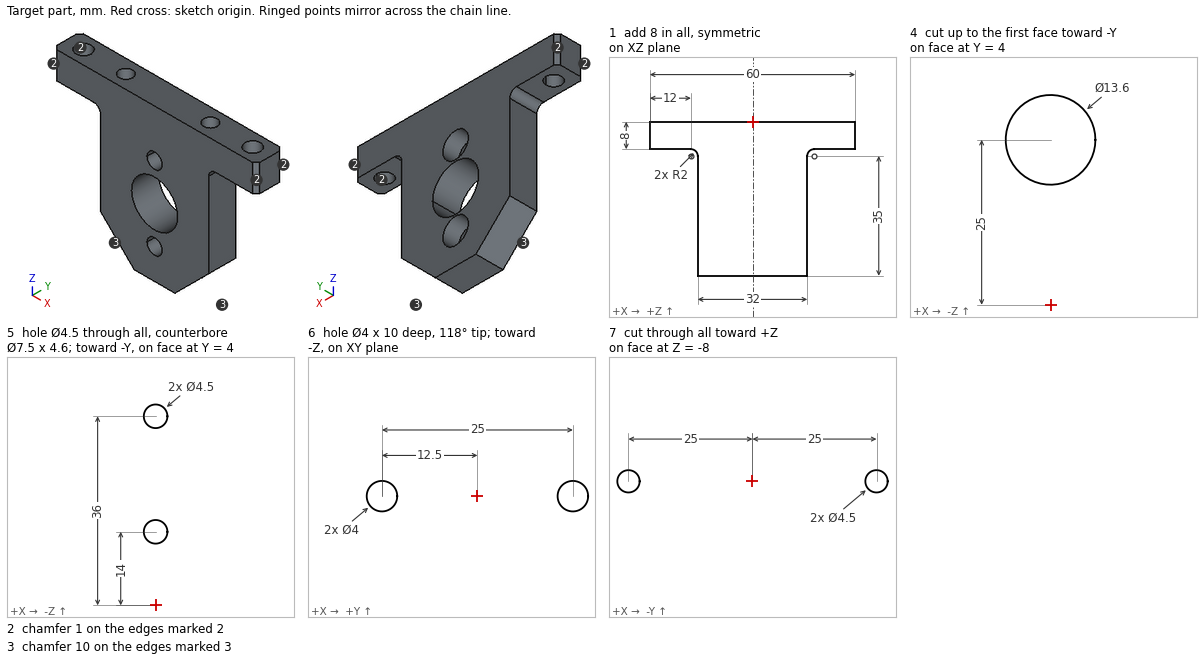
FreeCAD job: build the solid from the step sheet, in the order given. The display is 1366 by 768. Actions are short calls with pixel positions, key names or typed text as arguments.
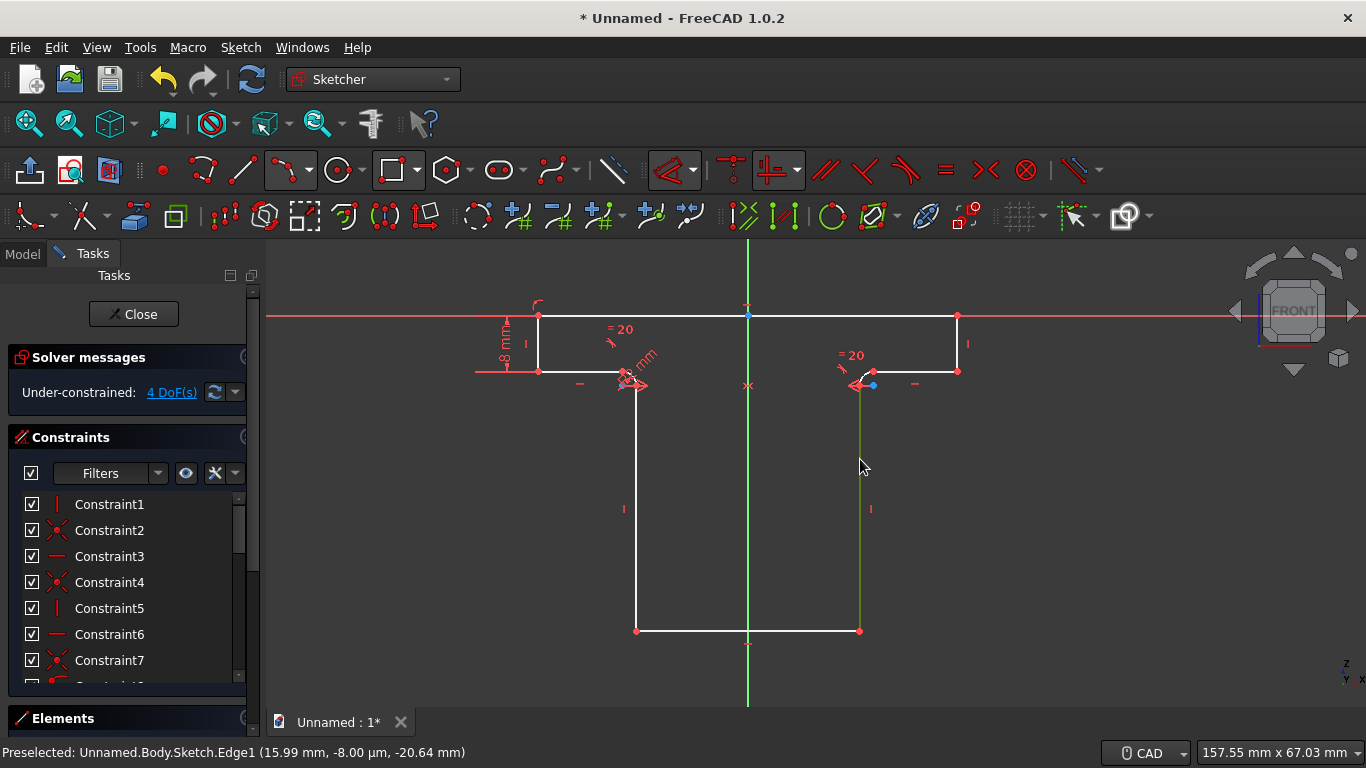
click(696, 170)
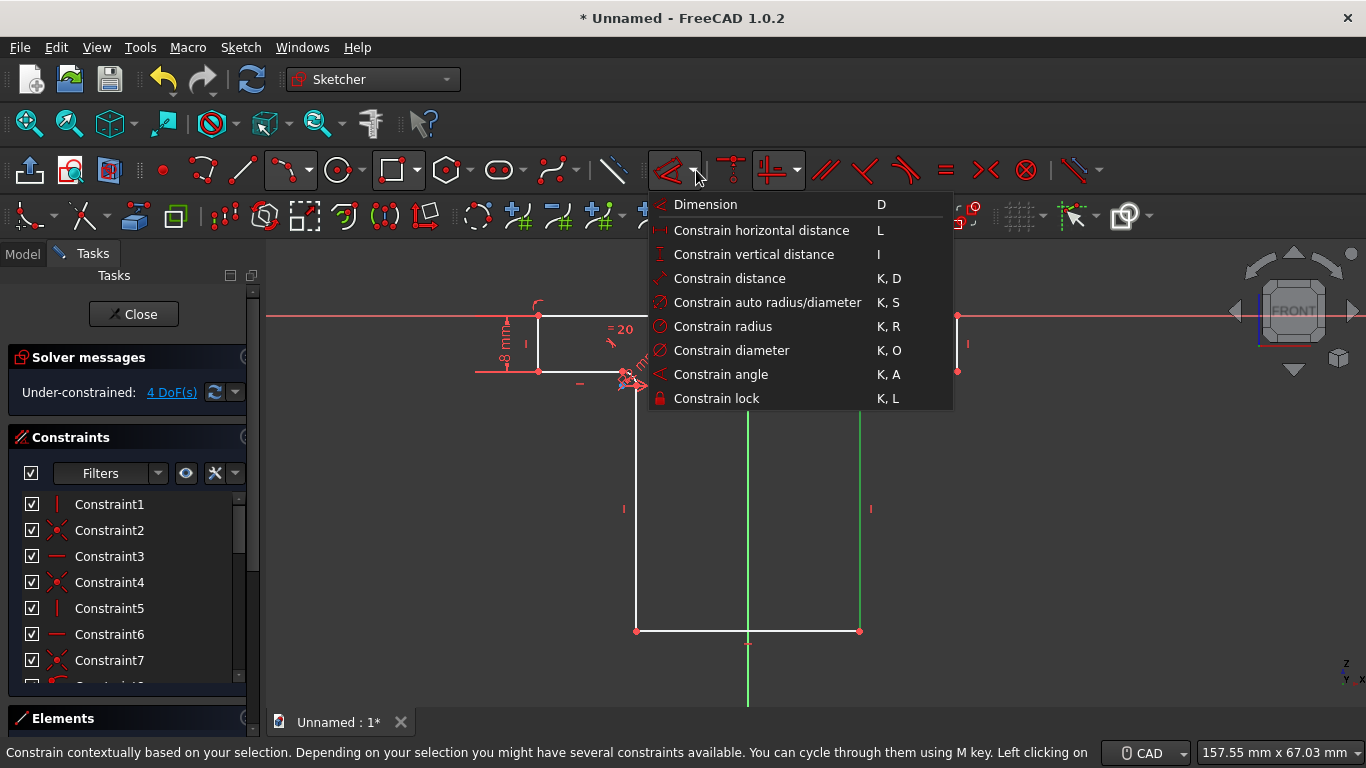
click(801, 254)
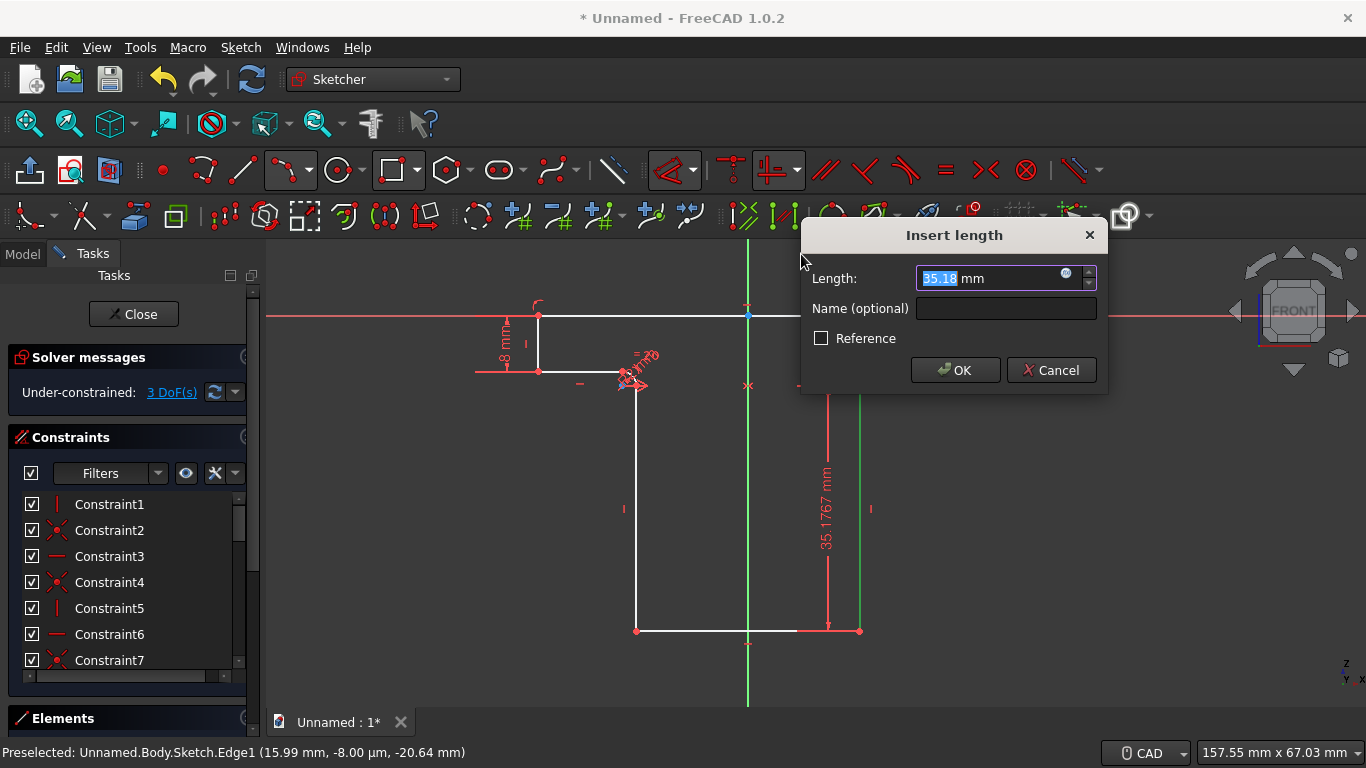
text(35)
key(Return)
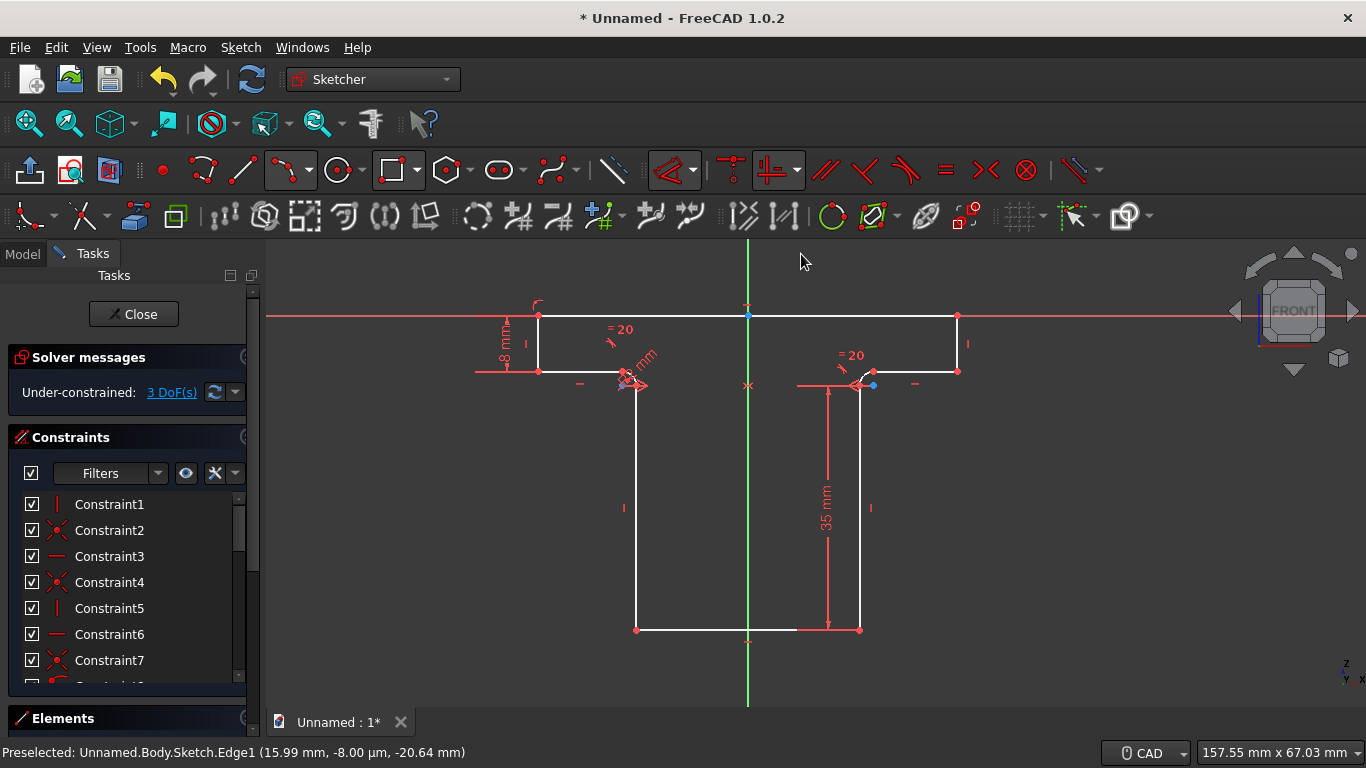
click(793, 630)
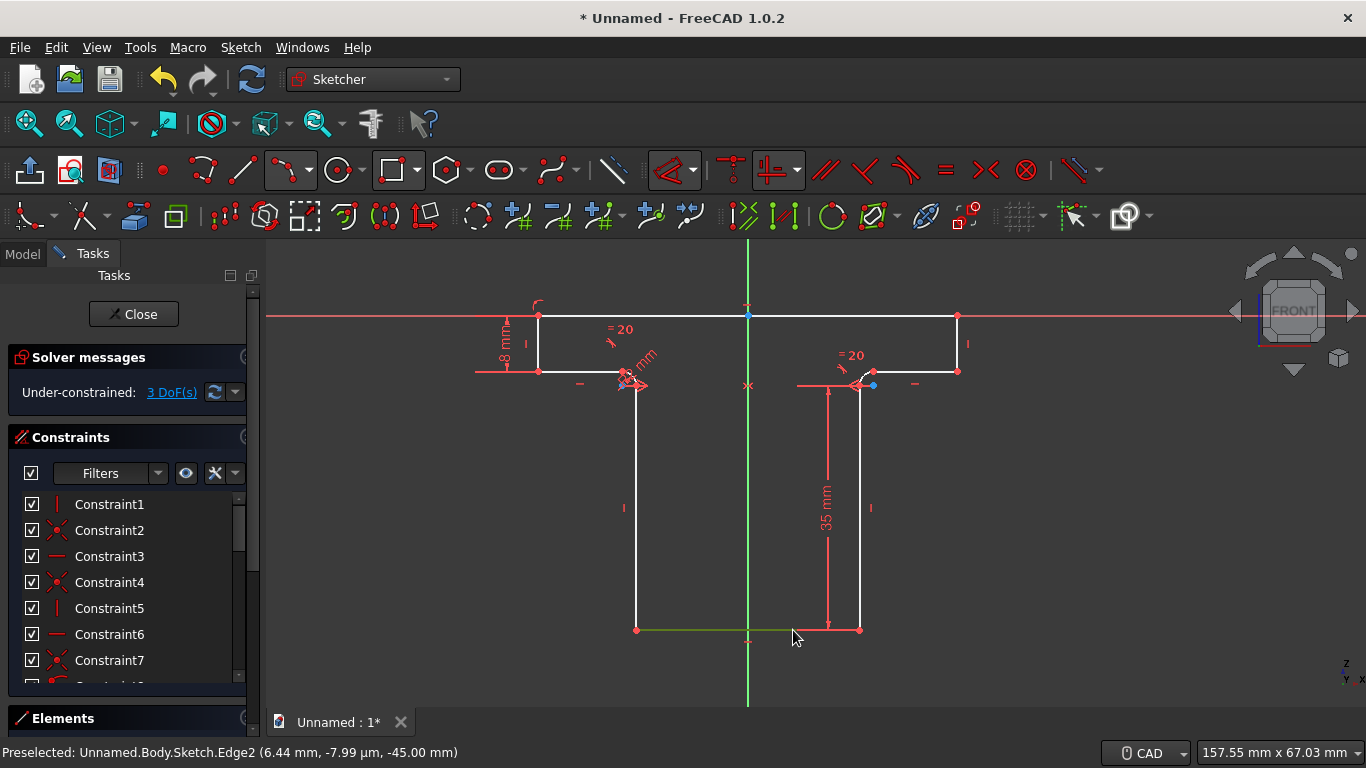
click(696, 170)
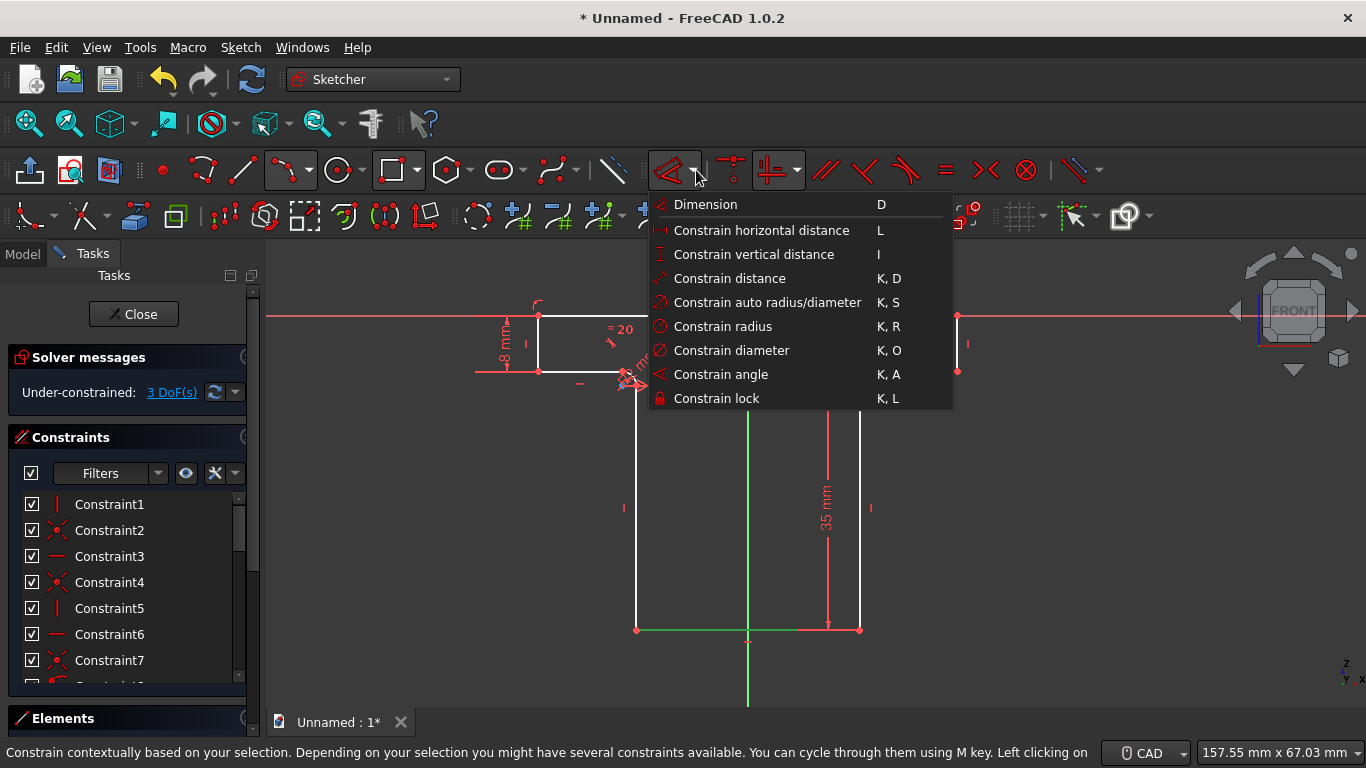
click(801, 230)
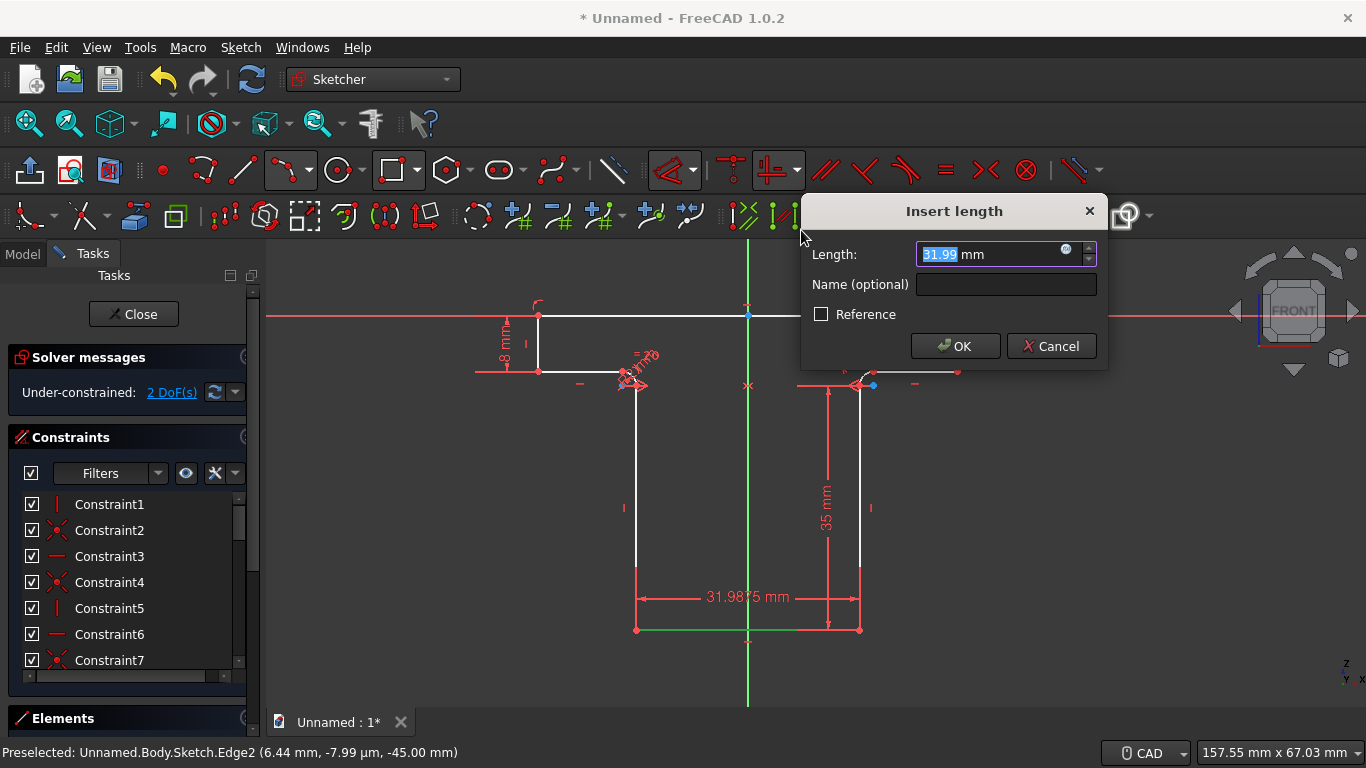
text(32)
key(Return)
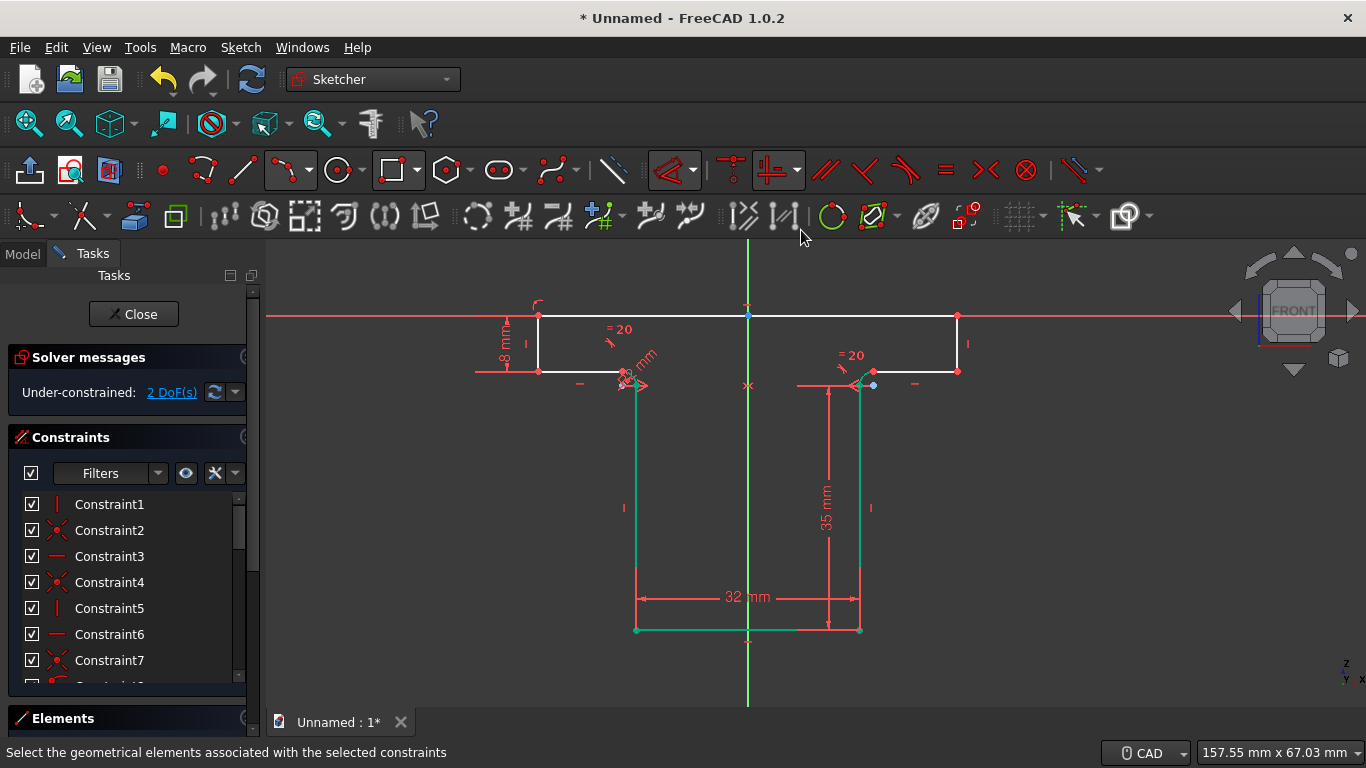
click(597, 372)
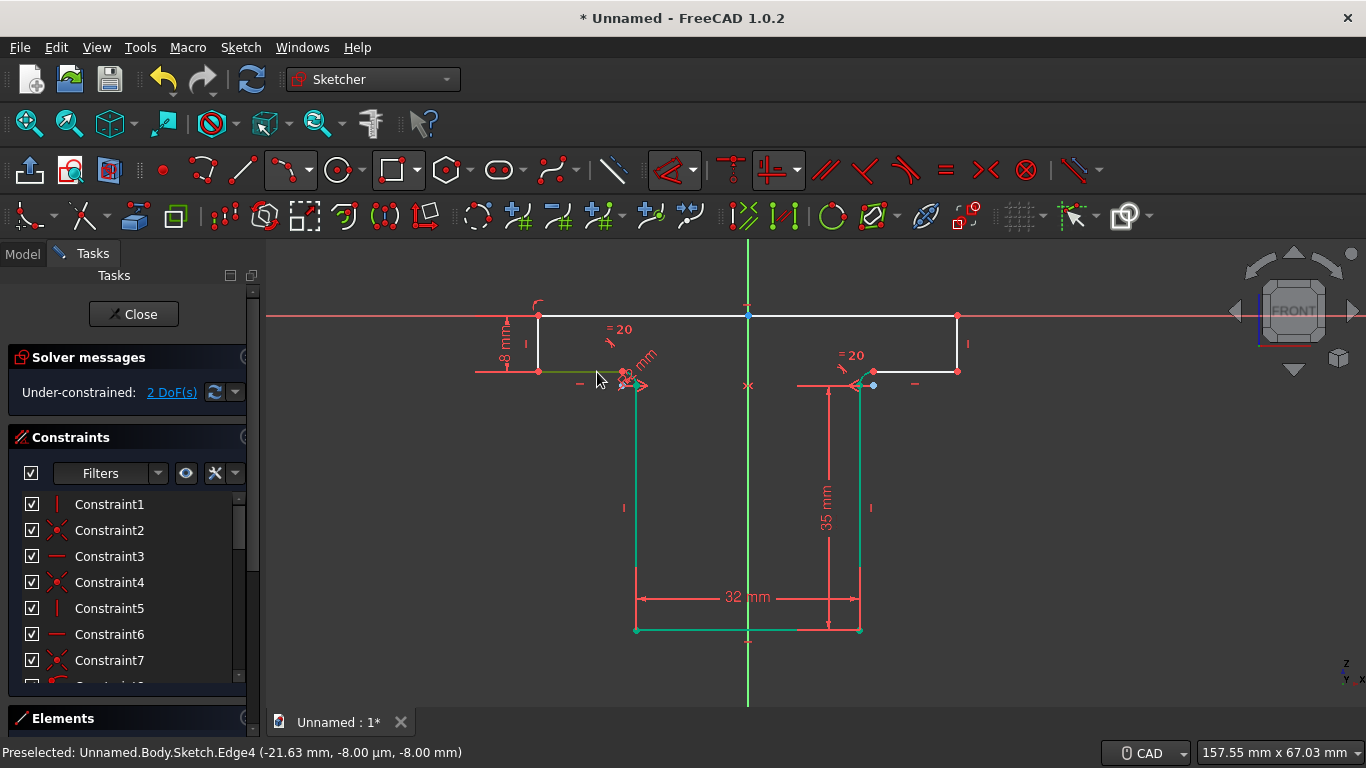
key(l)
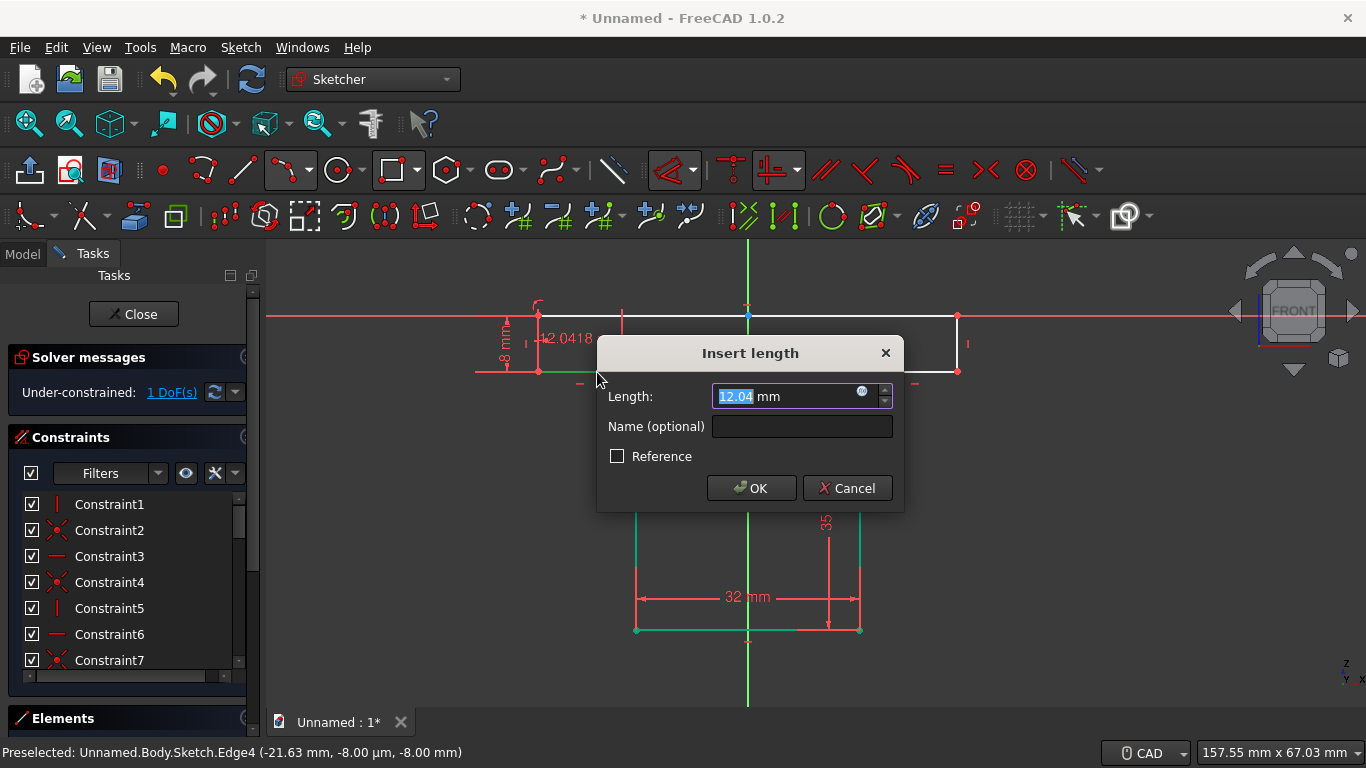
text(12)
key(Return)